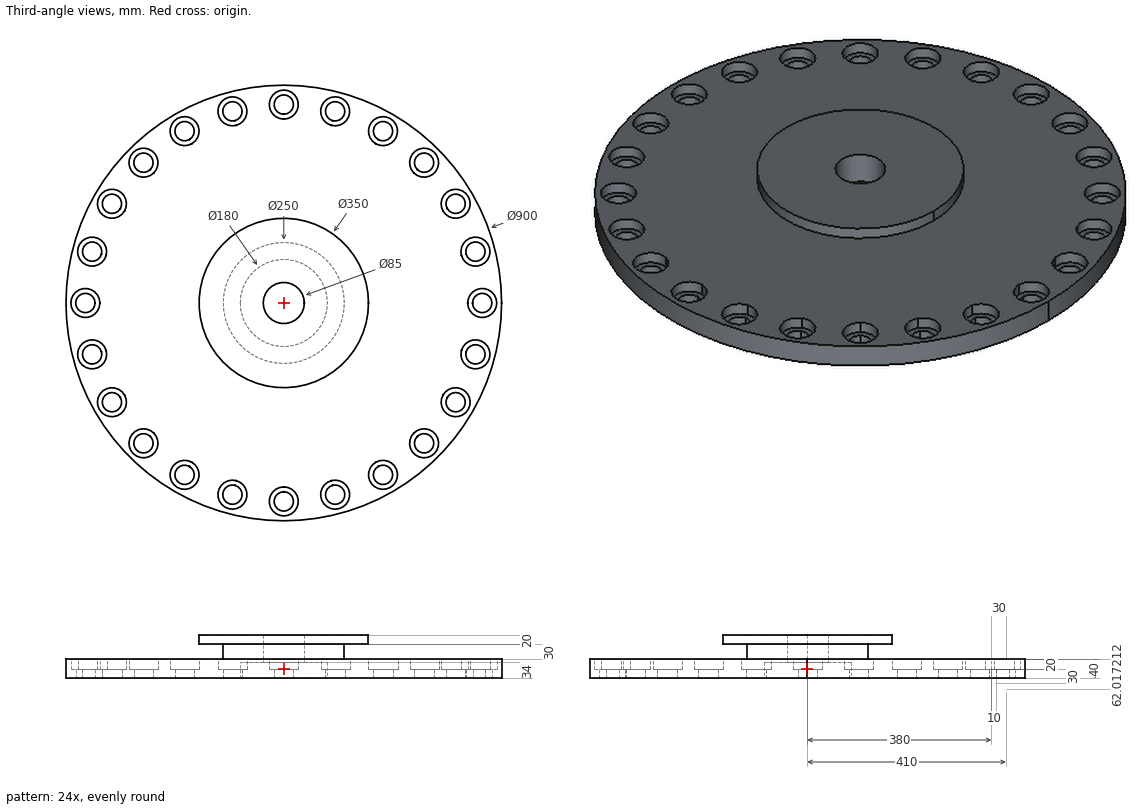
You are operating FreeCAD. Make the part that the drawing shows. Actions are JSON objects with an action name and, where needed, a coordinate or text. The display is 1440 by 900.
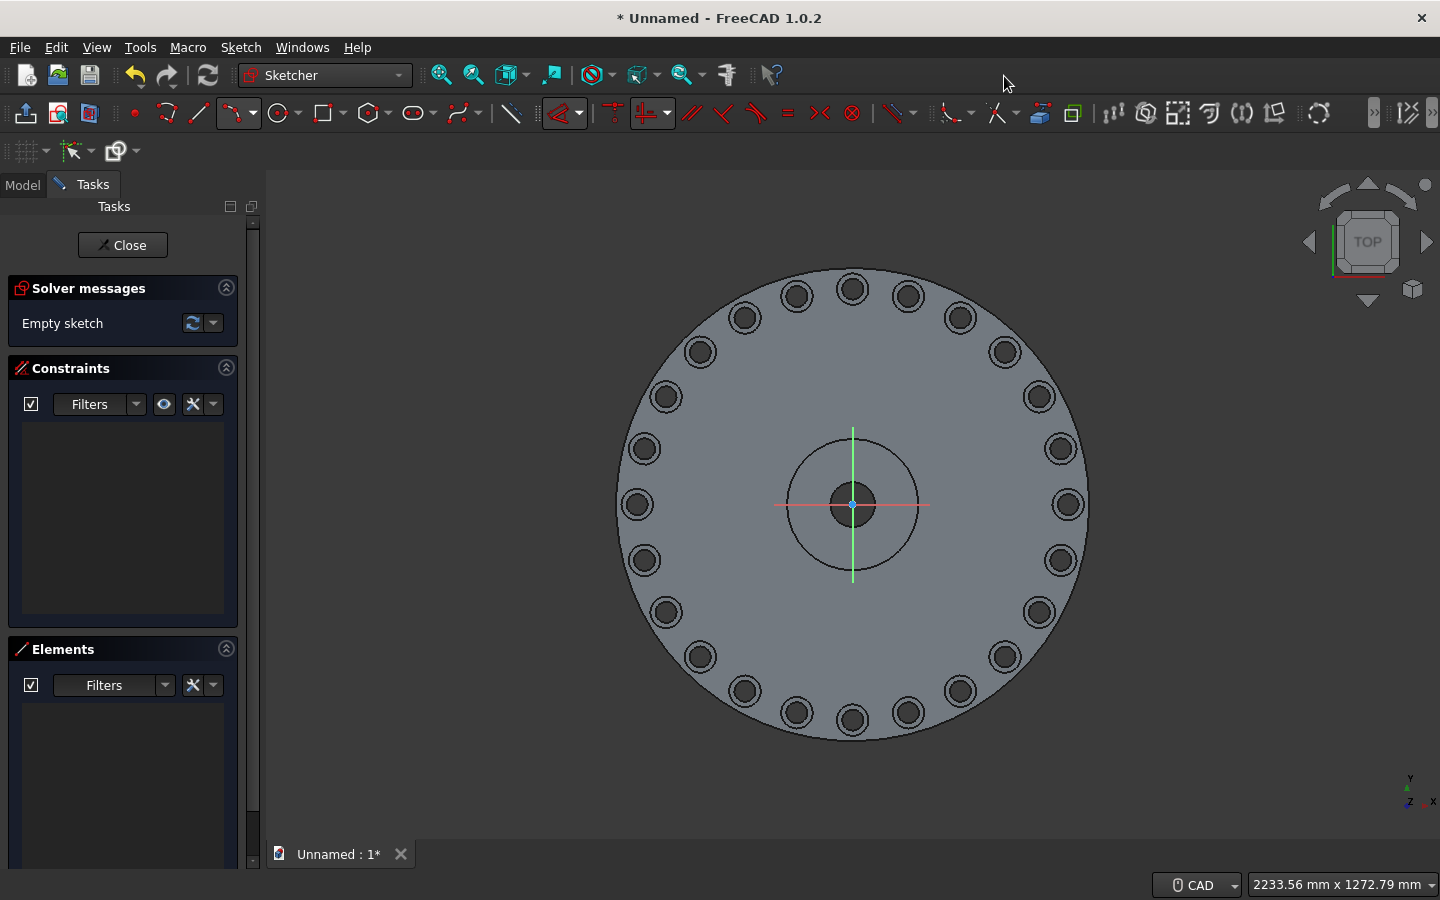
{"action": "scroll", "coordinate": [908, 505], "scroll_direction": "up", "scroll_amount": 4}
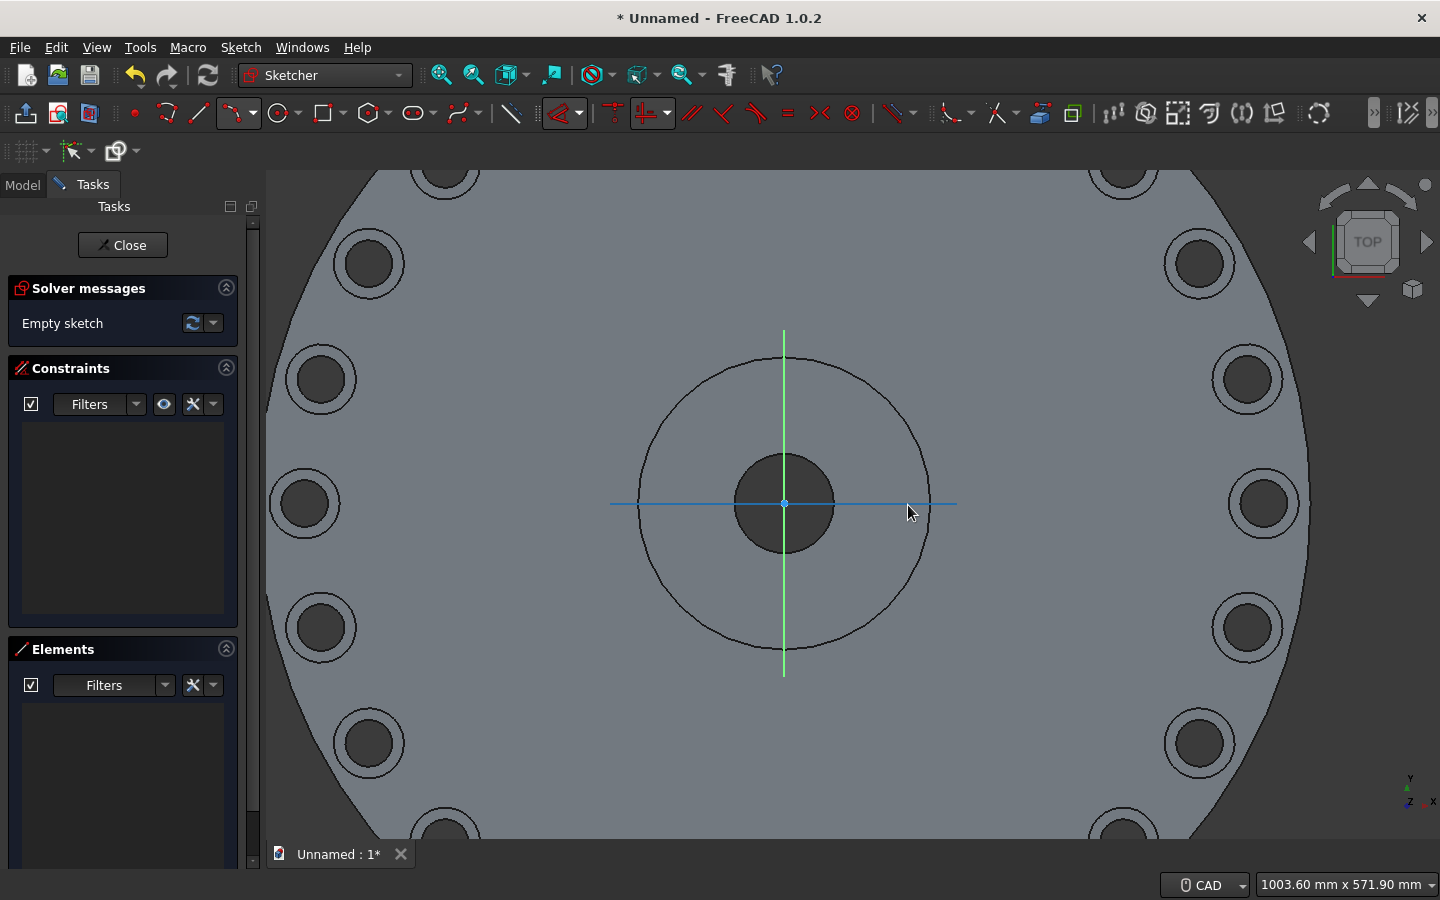
{"action": "left_click", "coordinate": [278, 114]}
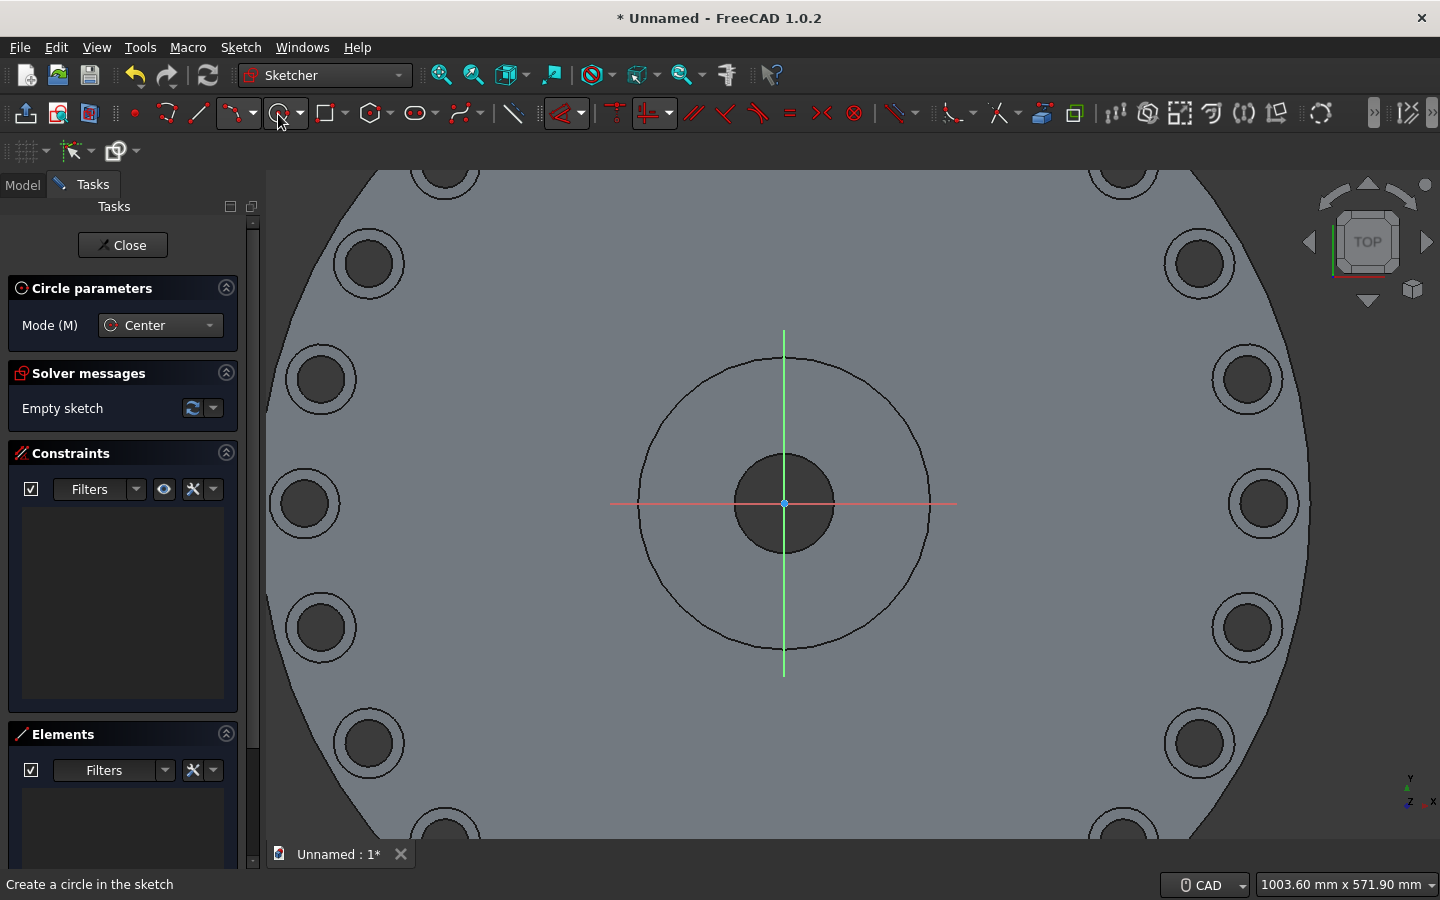
{"action": "left_click", "coordinate": [784, 504]}
{"action": "mouse_move", "coordinate": [929, 359]}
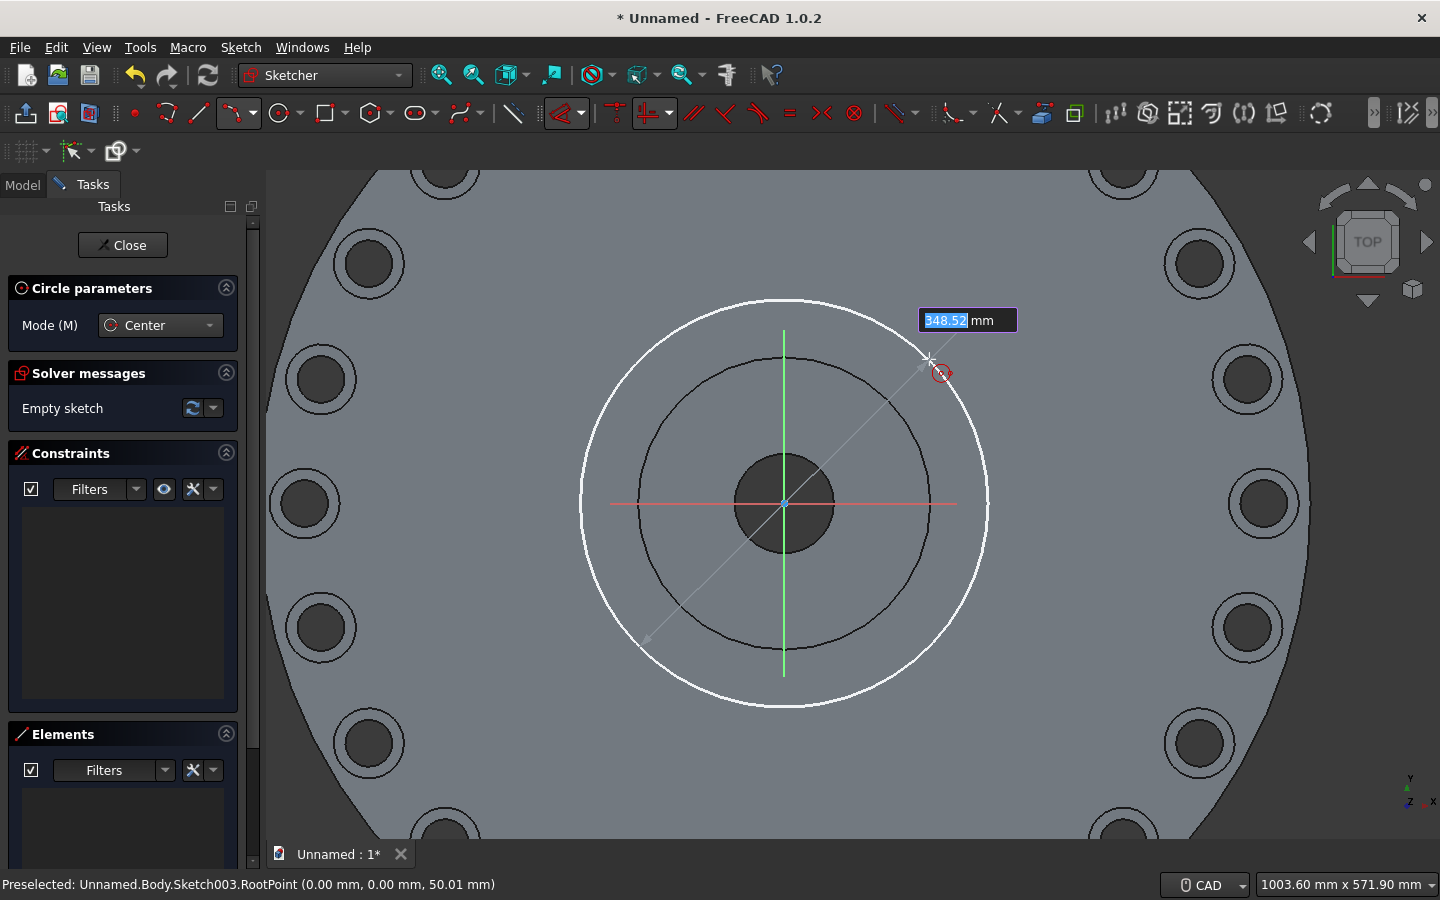
{"action": "type", "text": "350"}
{"action": "key", "text": "Return"}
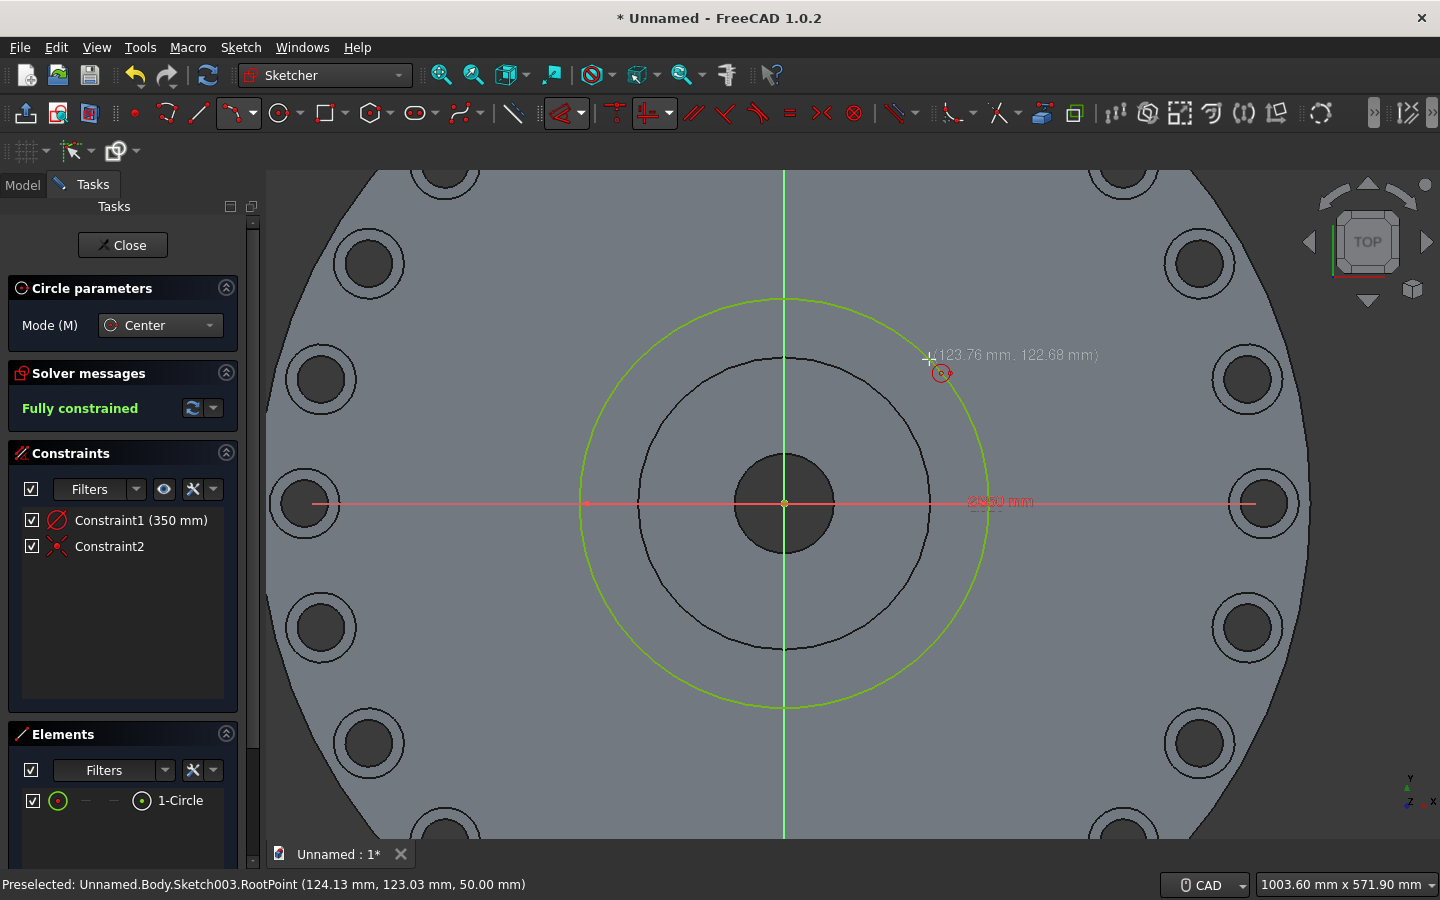
{"action": "left_click", "coordinate": [784, 504]}
{"action": "mouse_move", "coordinate": [819, 468]}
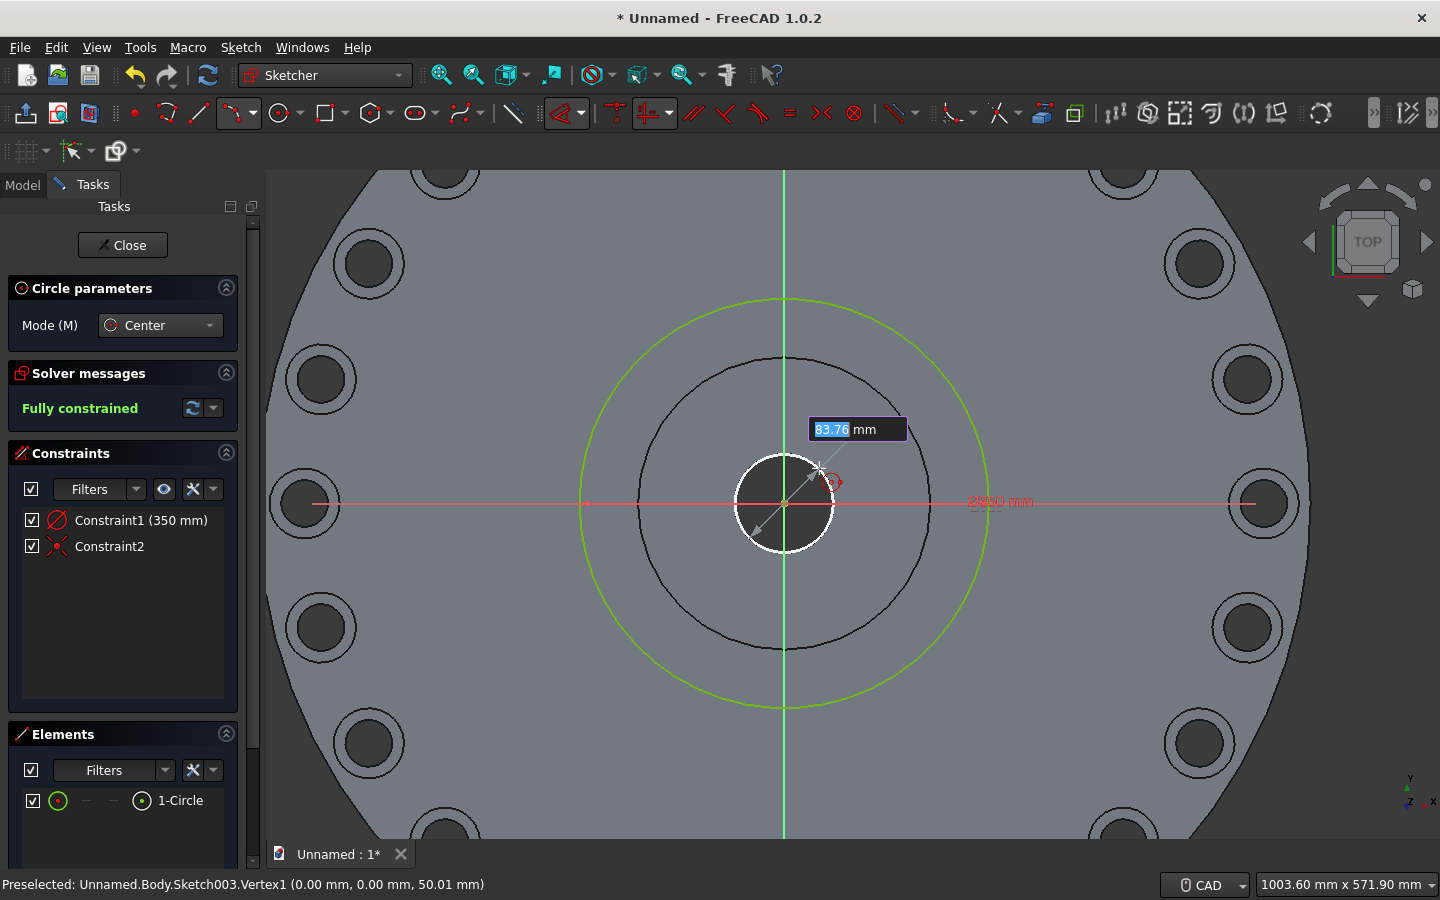
{"action": "type", "text": "85"}
{"action": "key", "text": "Return"}
{"action": "key", "text": "Escape"}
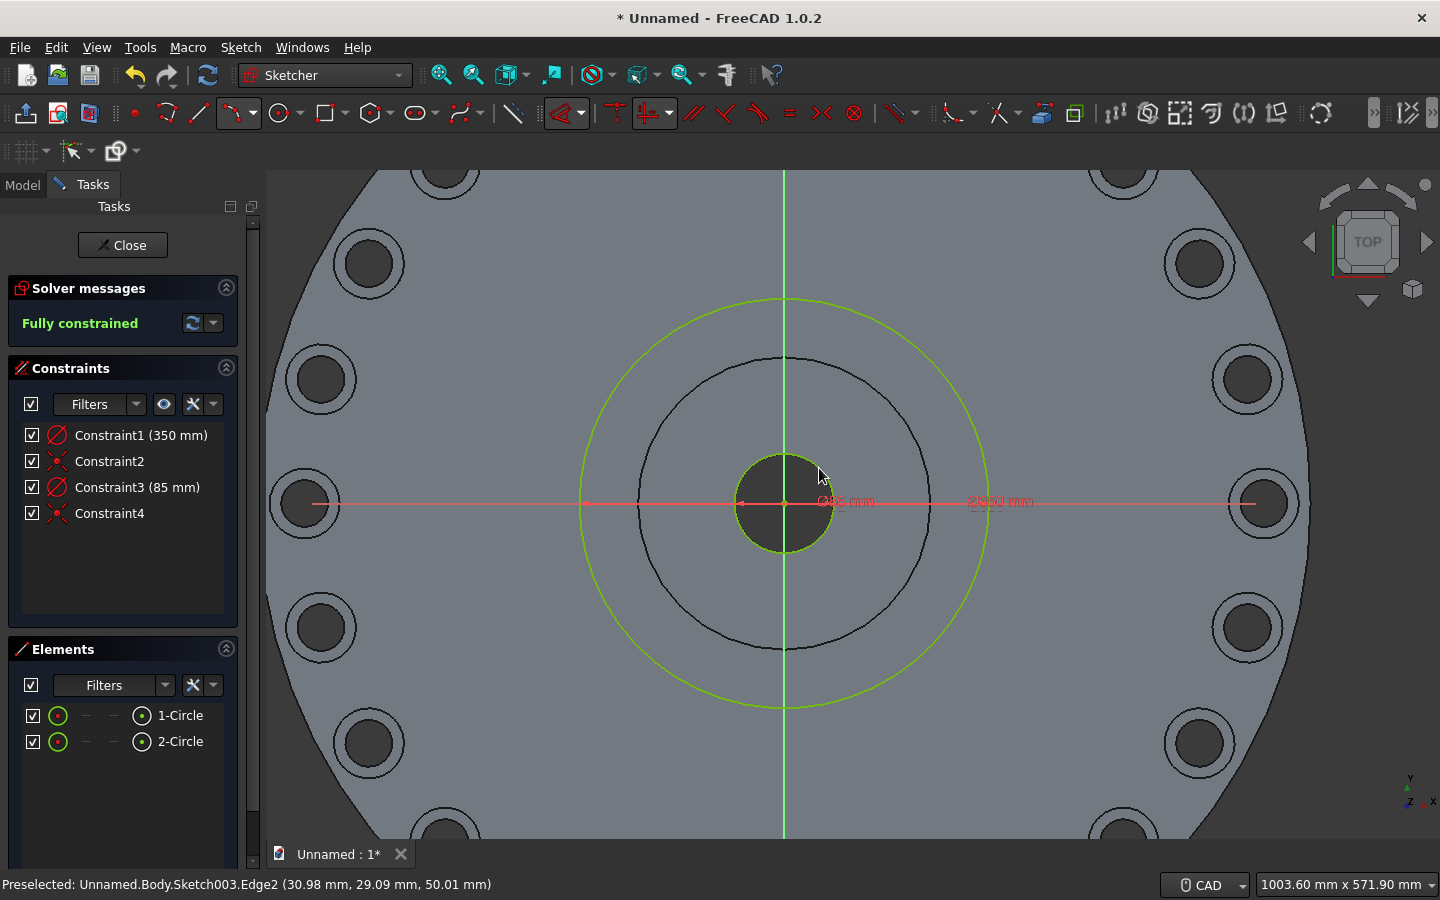
{"action": "left_click", "coordinate": [123, 245]}